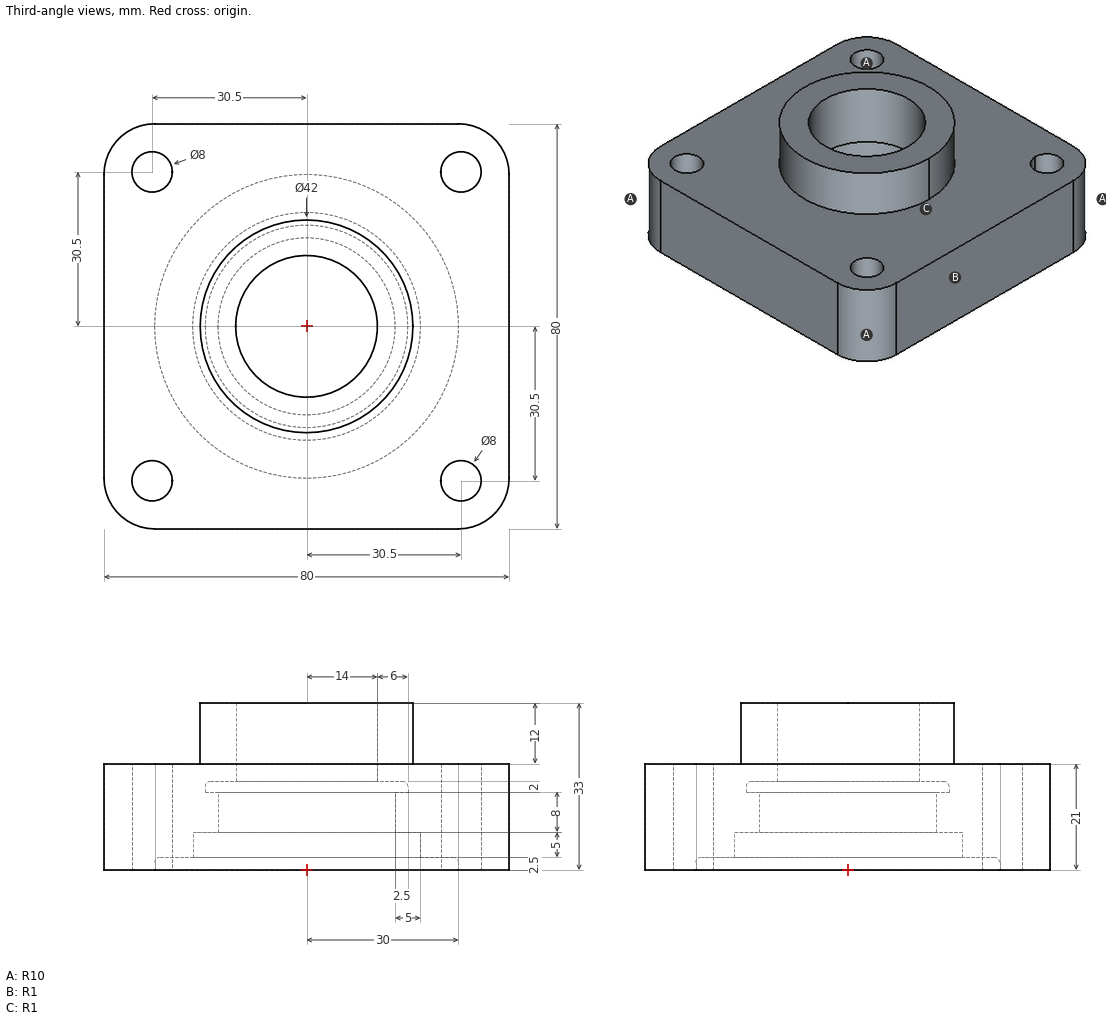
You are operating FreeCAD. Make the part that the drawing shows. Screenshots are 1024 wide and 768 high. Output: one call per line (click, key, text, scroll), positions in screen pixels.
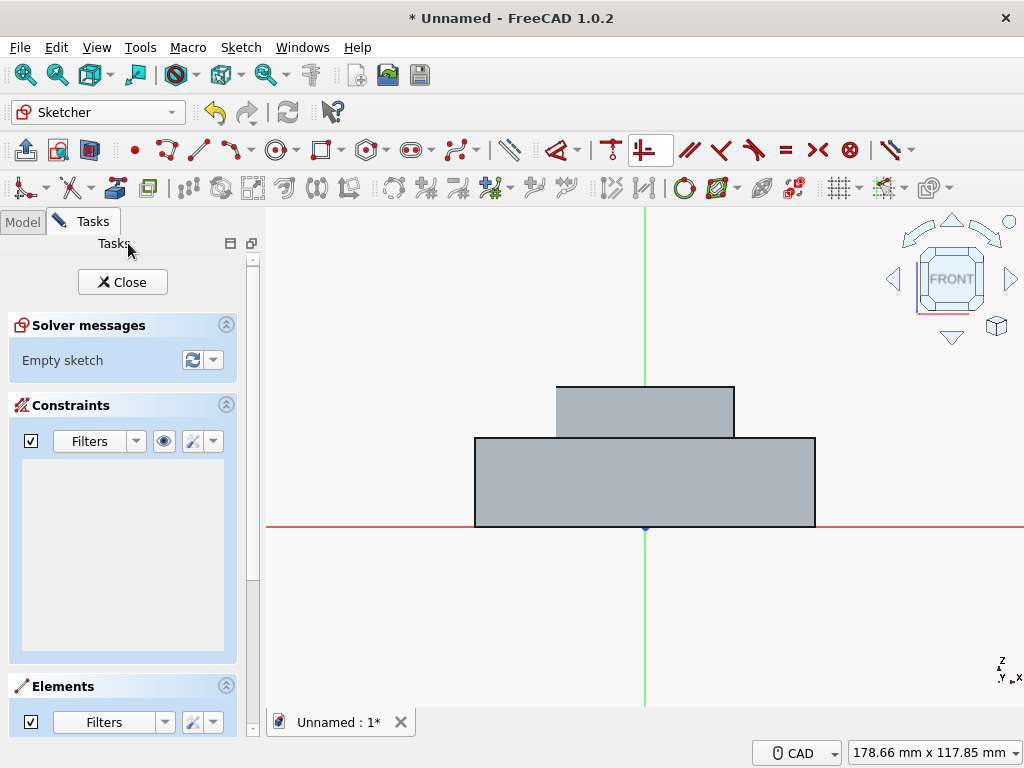
click(90, 150)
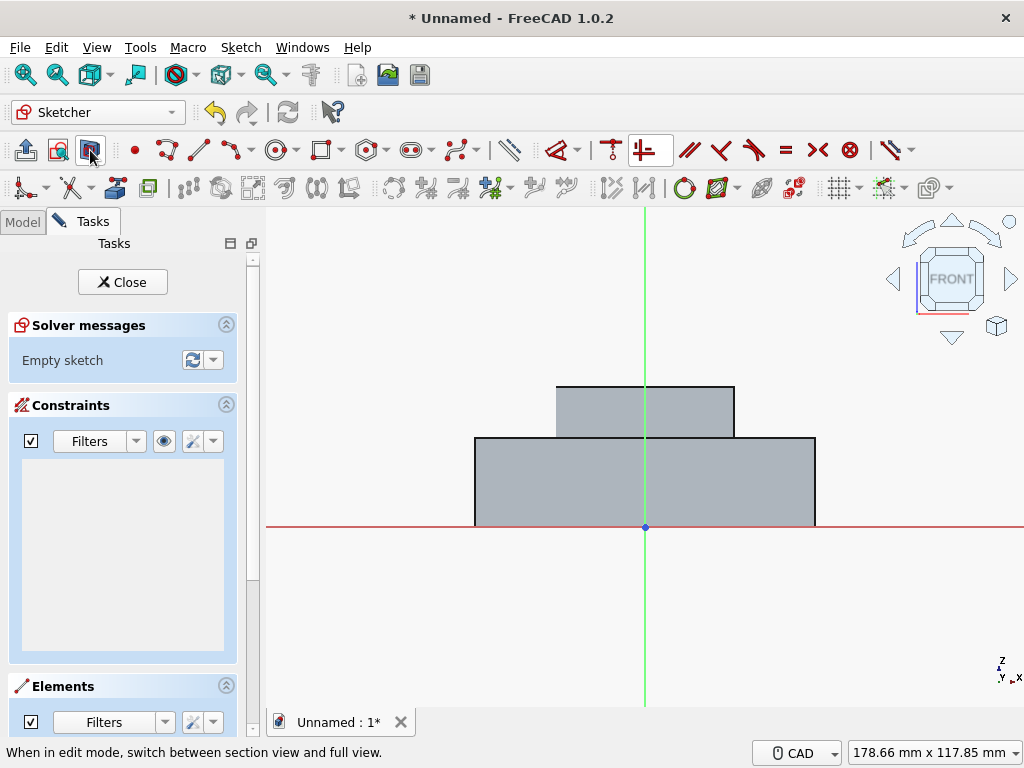
scroll(816, 457, up, 4)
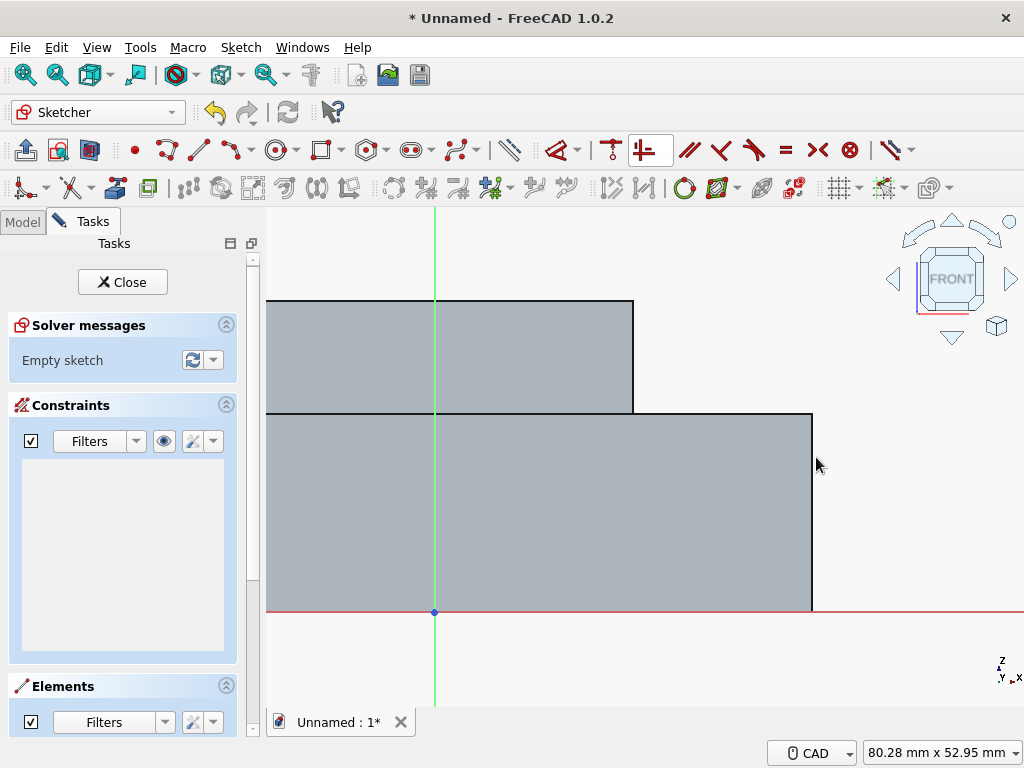
click(168, 150)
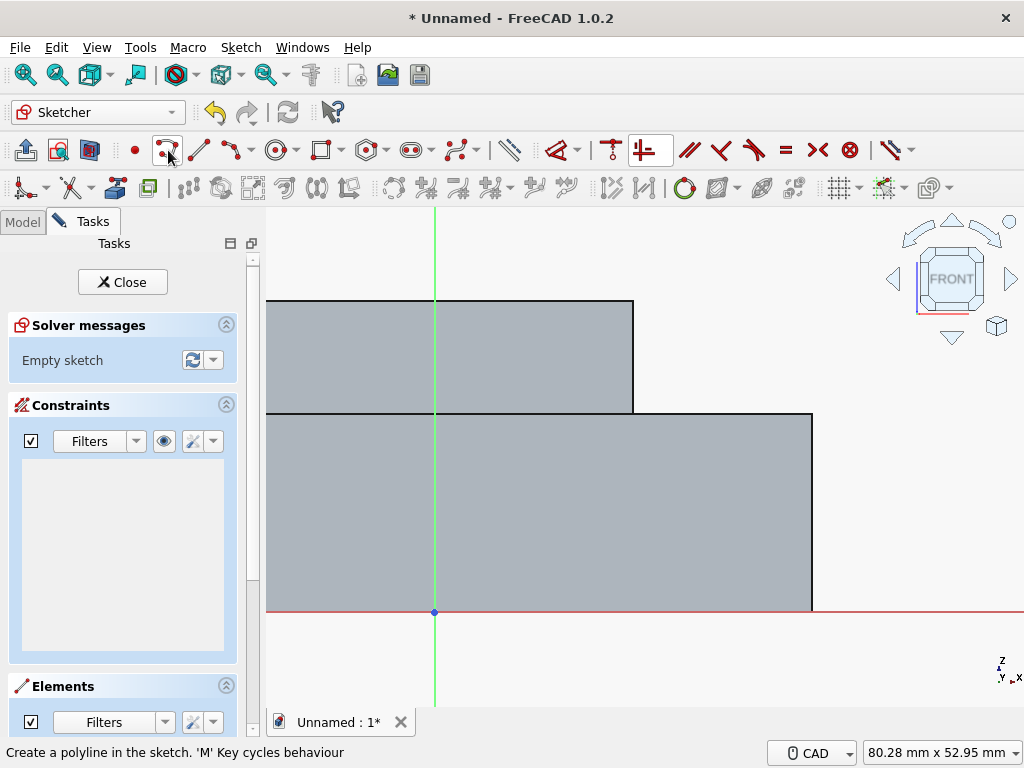
click(435, 612)
click(444, 301)
click(567, 301)
click(567, 447)
click(623, 447)
click(623, 466)
click(600, 466)
click(600, 541)
click(647, 541)
click(647, 589)
click(718, 589)
click(718, 603)
click(435, 612)
key(Escape)
key(Escape)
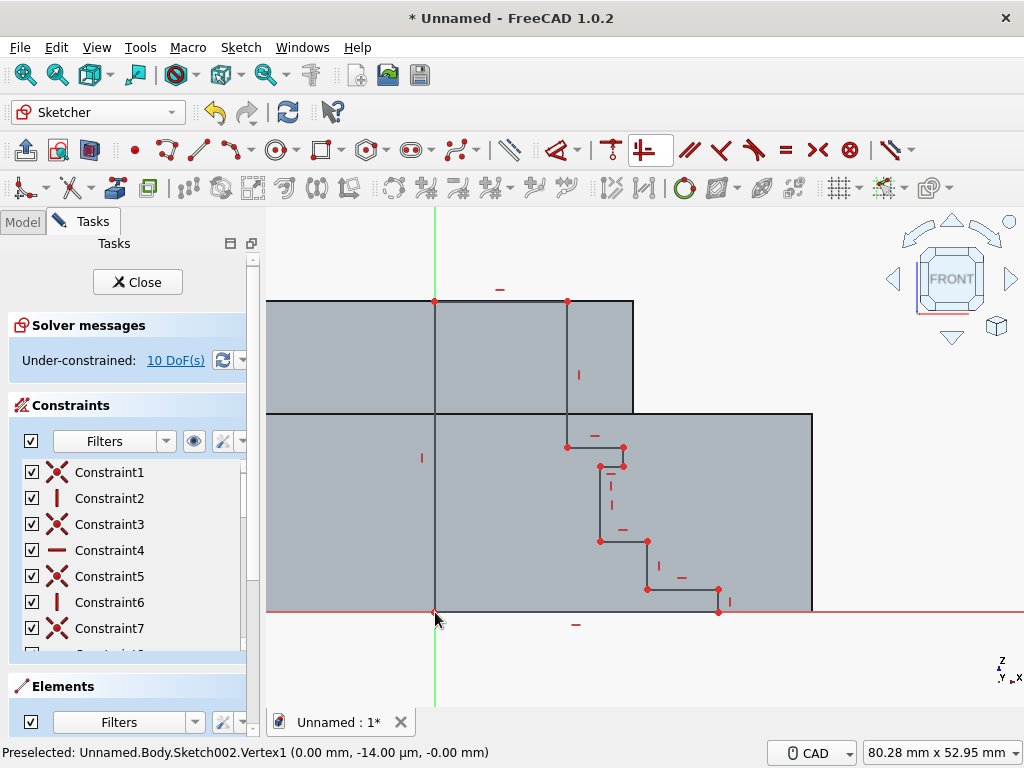
click(584, 448)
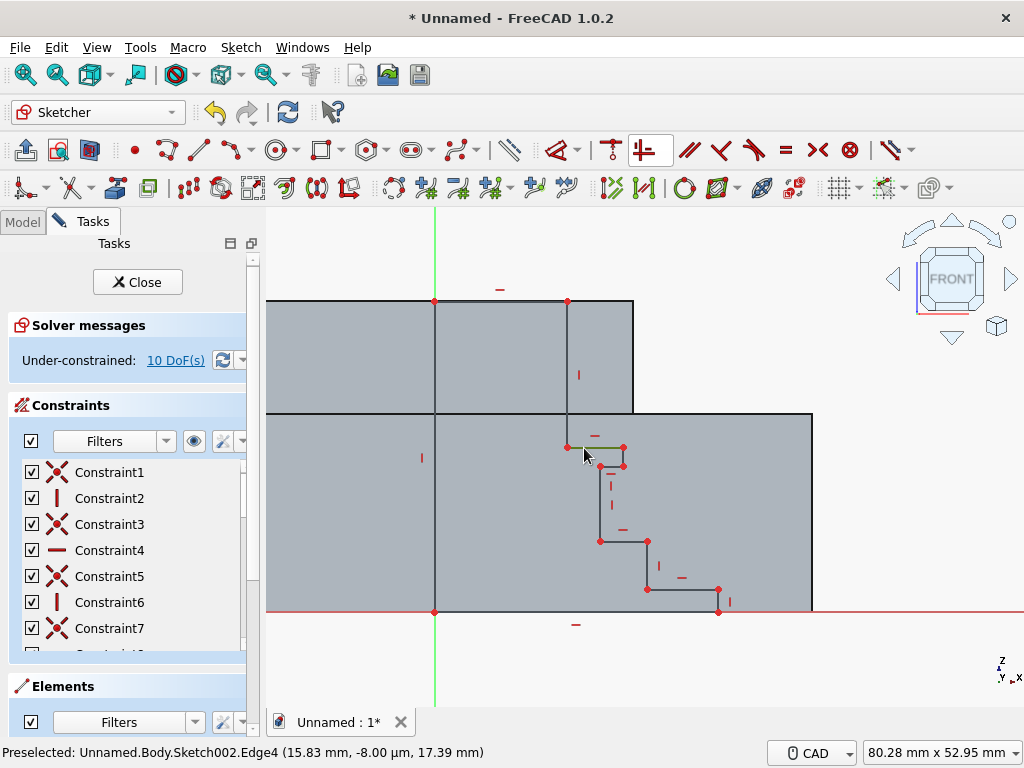
click(580, 150)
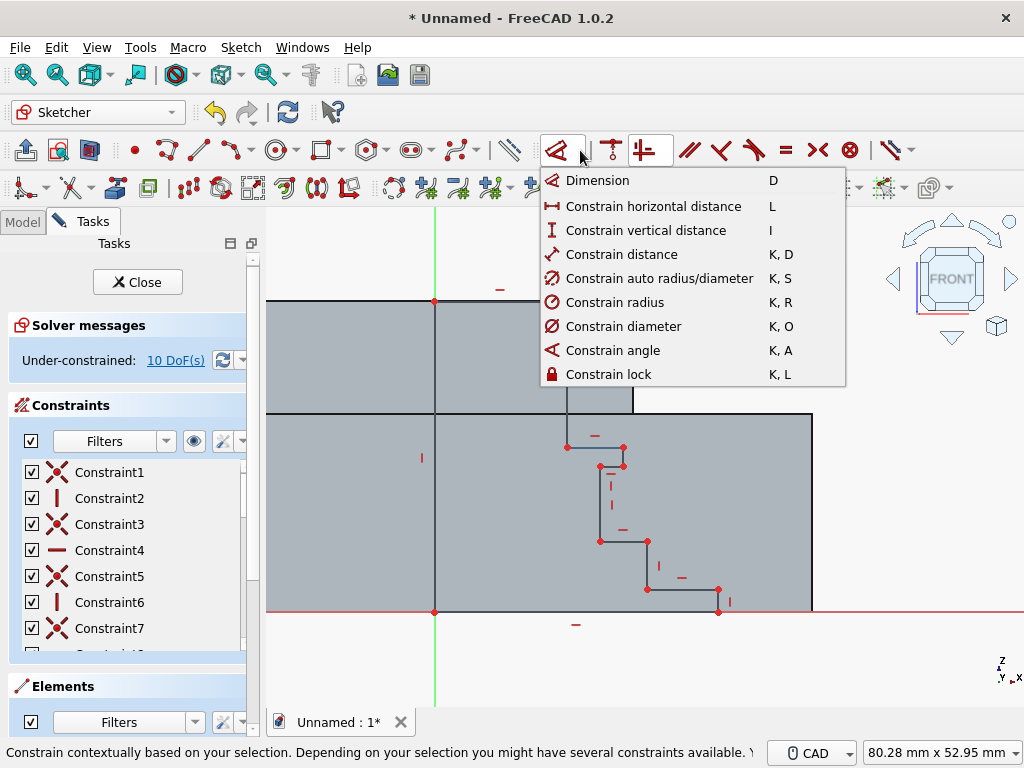
click(693, 206)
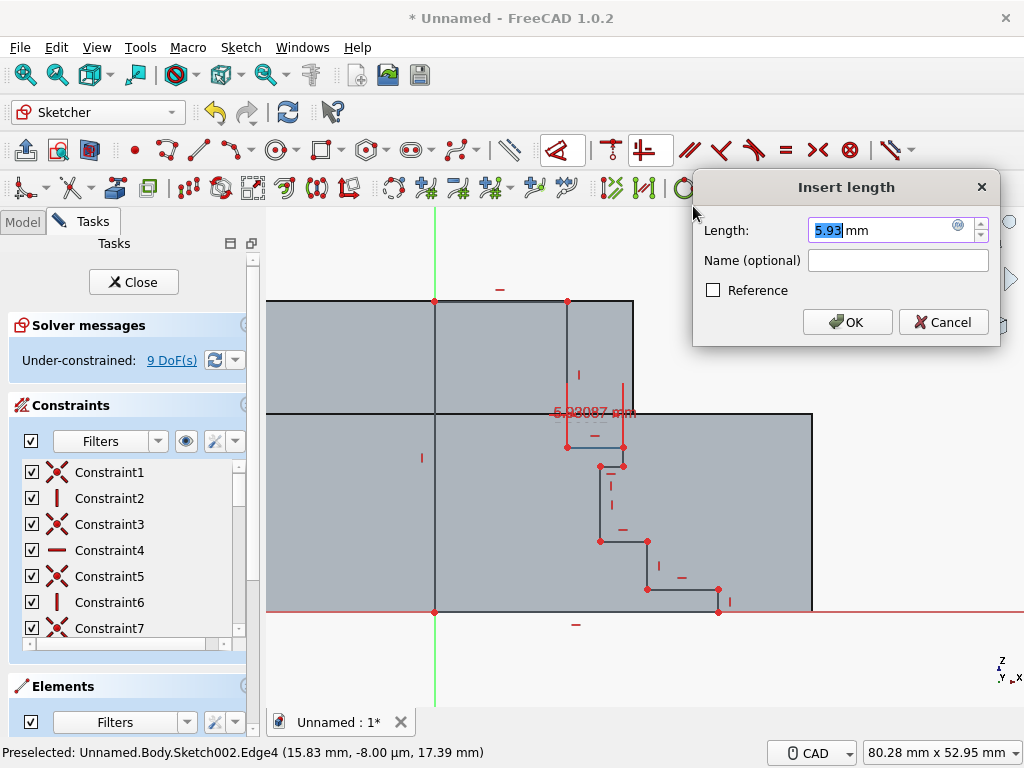
text(6)
key(Return)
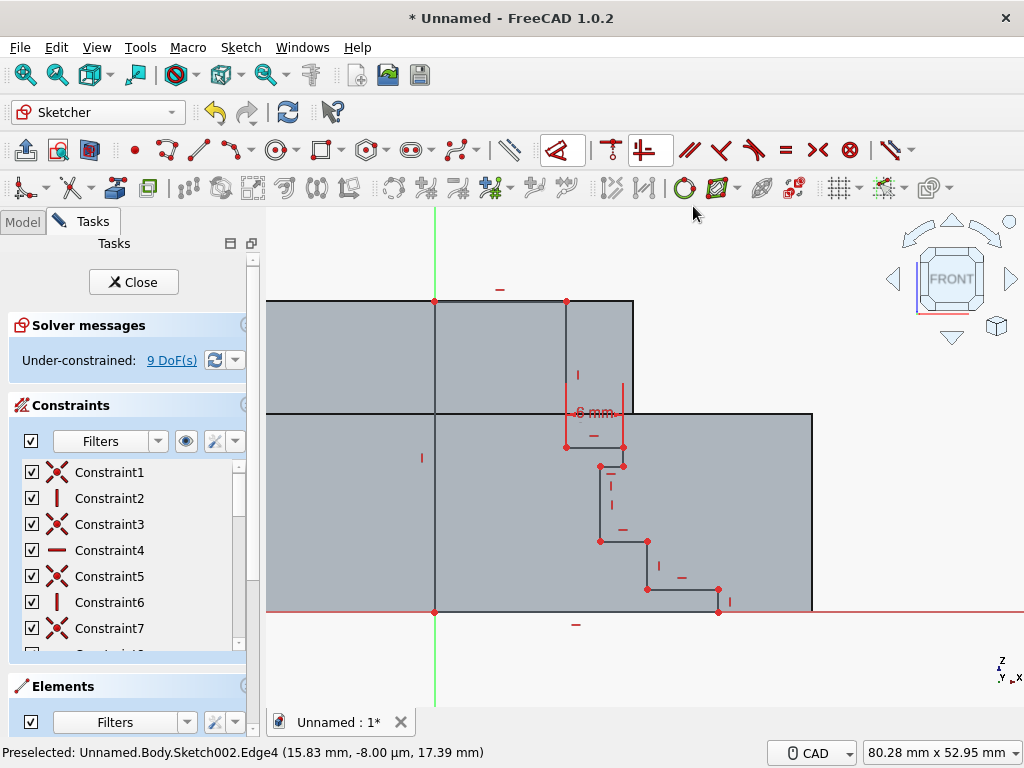
scroll(623, 458, up, 4)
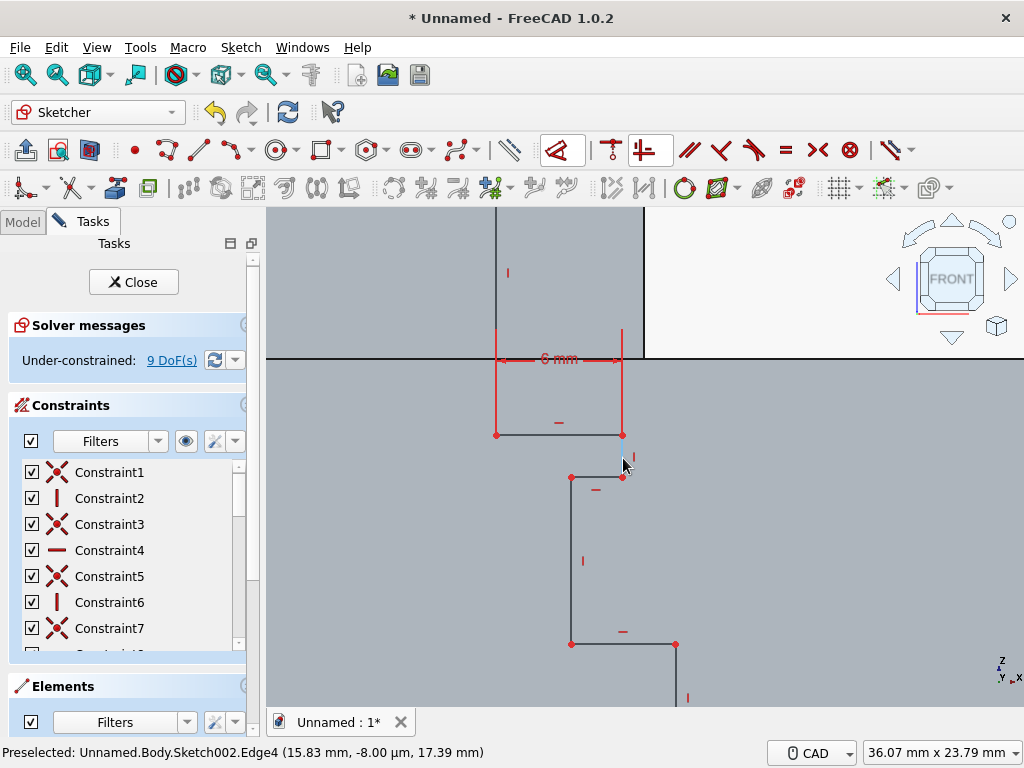
click(622, 456)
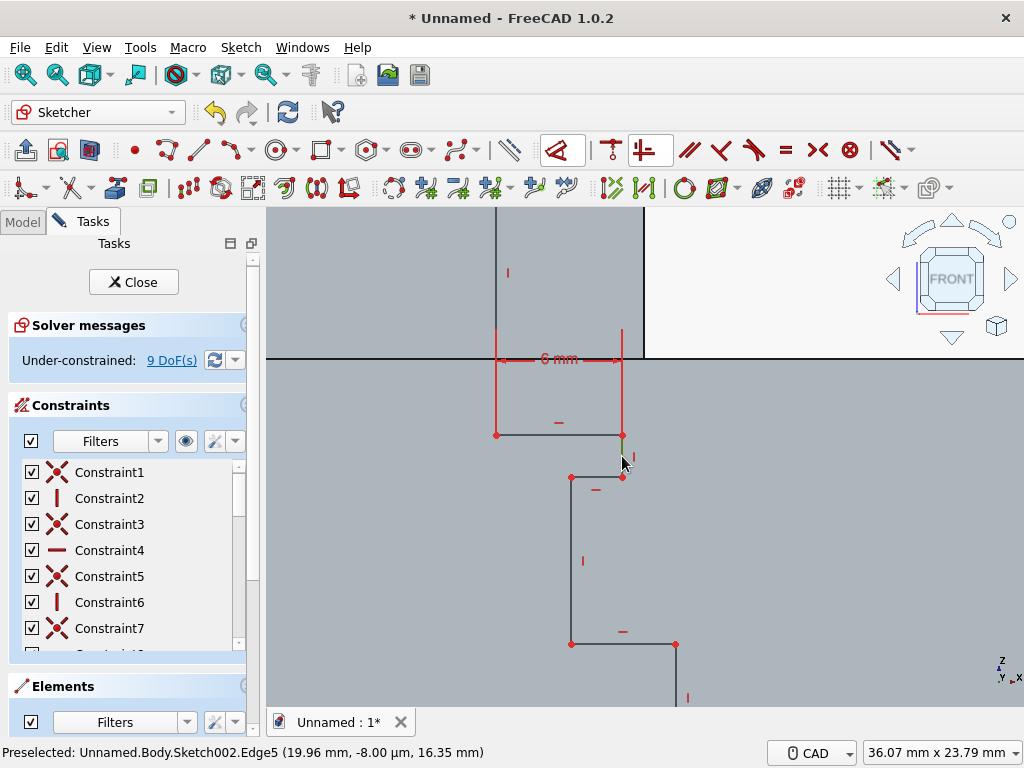
key(i)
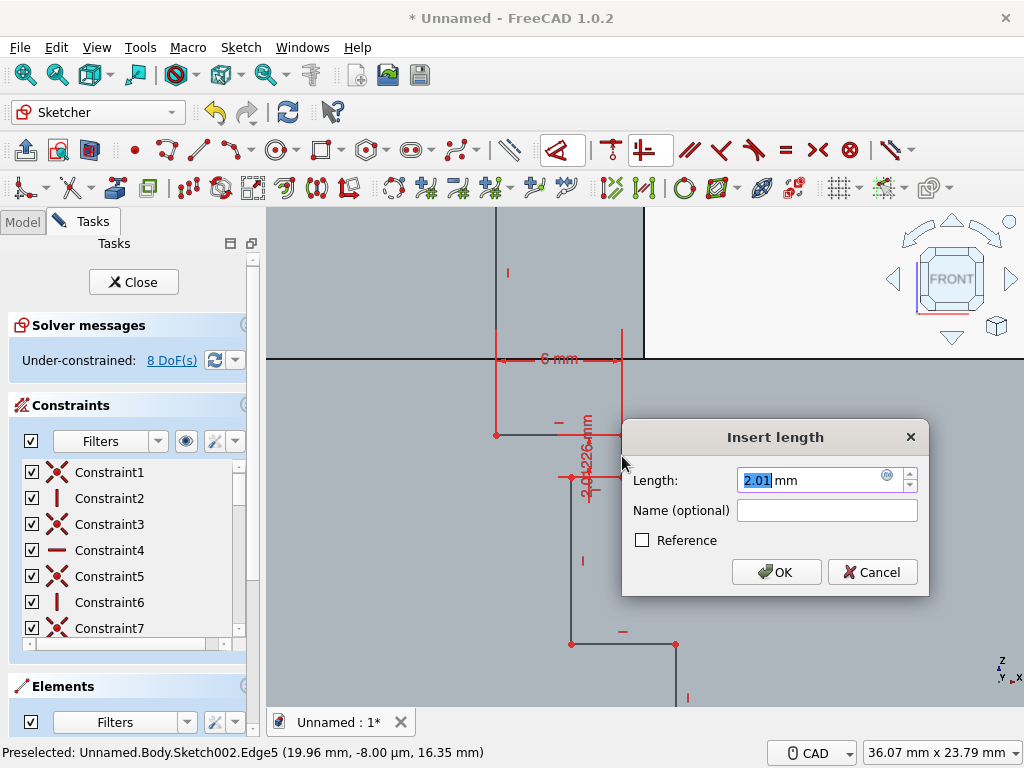
text(2)
key(Return)